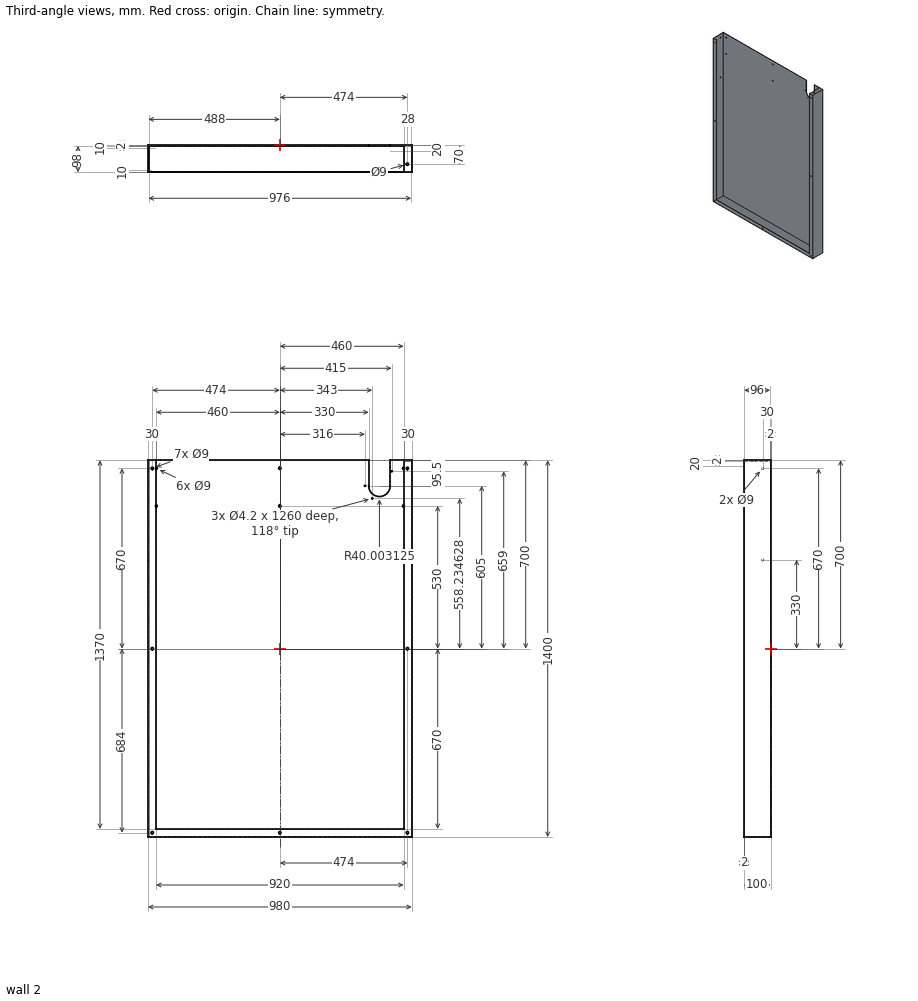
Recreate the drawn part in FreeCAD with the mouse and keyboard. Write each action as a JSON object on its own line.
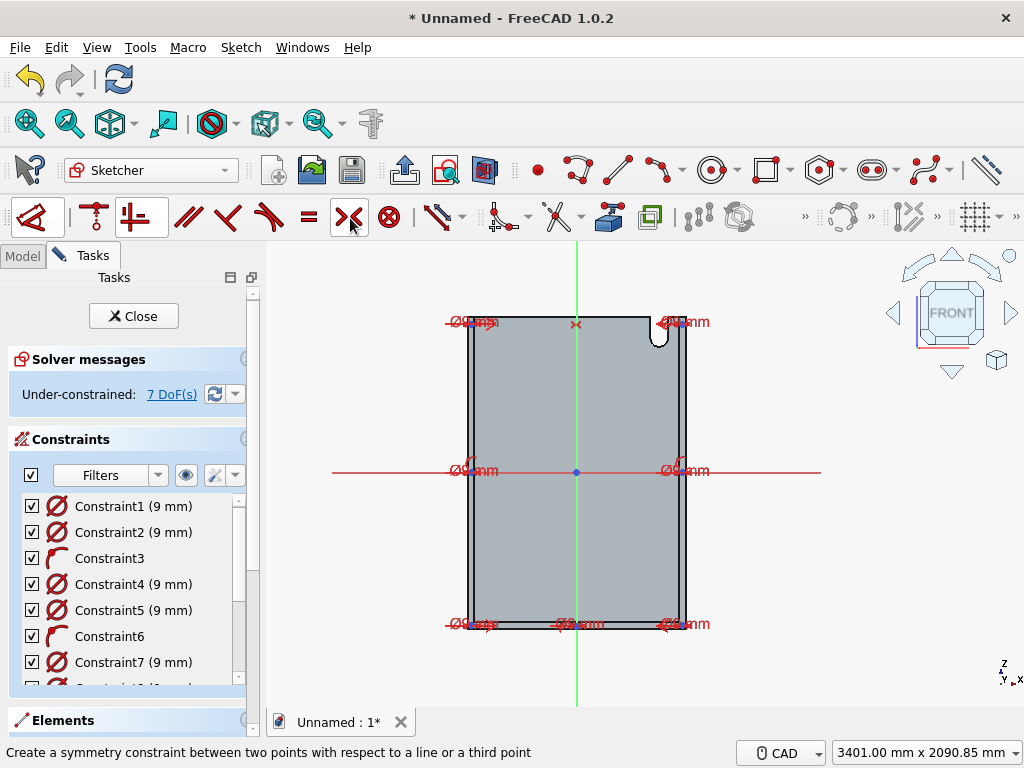
{"action": "left_click", "coordinate": [471, 324]}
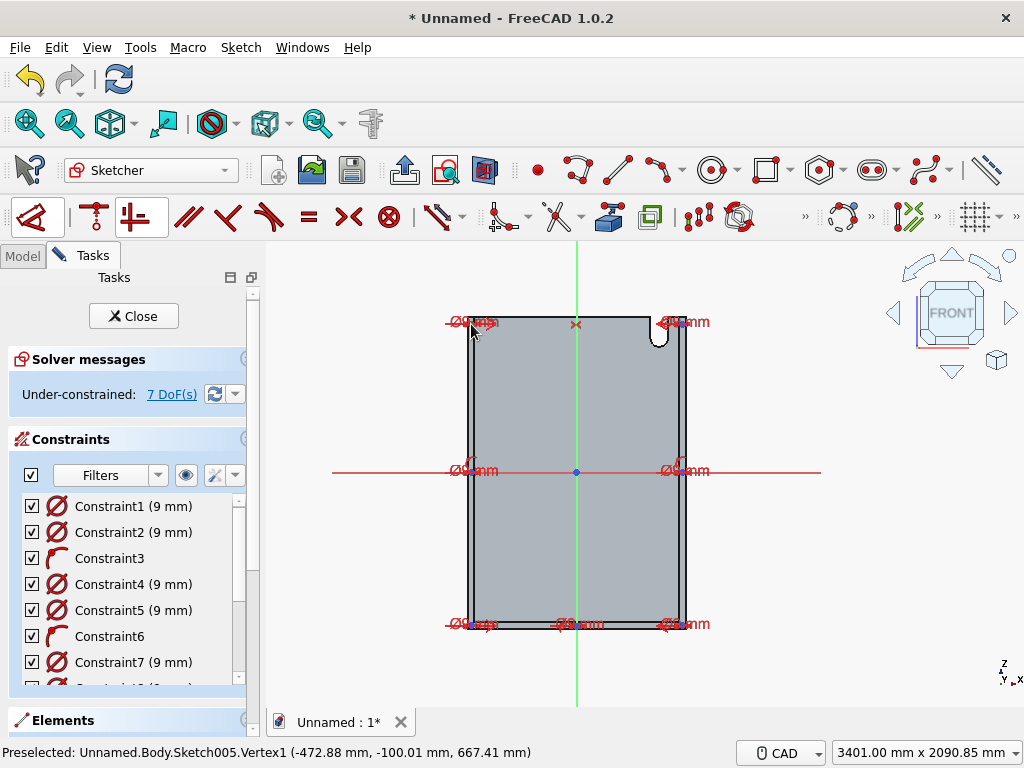
{"action": "key", "text": "l"}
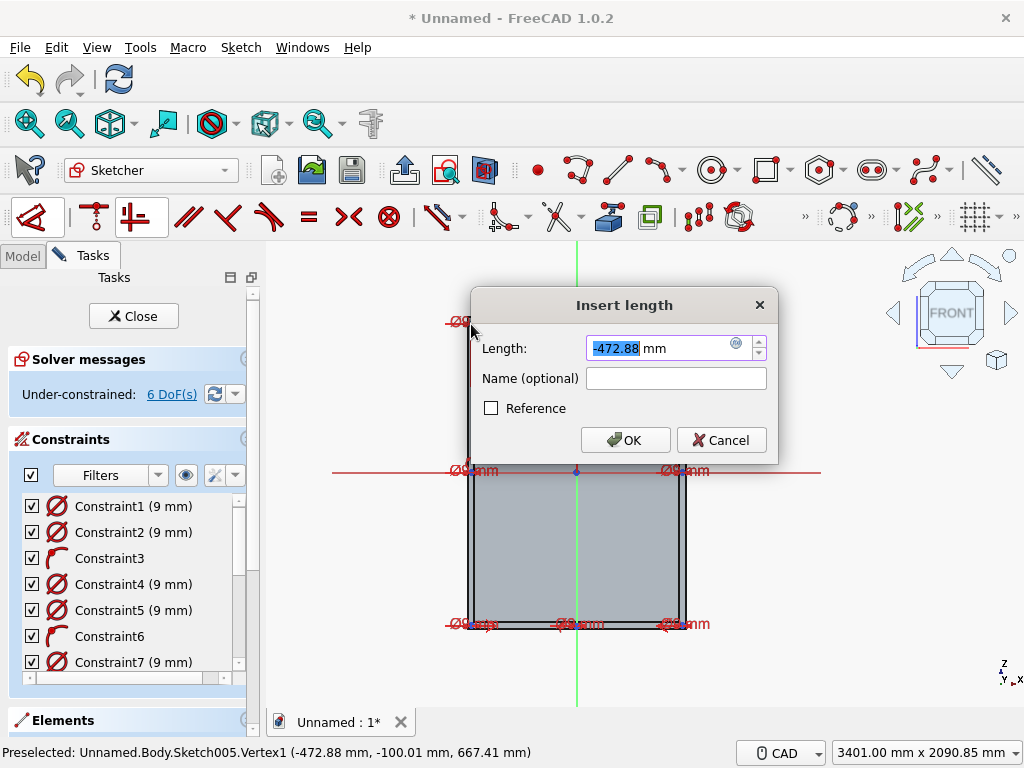
{"action": "type", "text": "-474"}
{"action": "key", "text": "Return"}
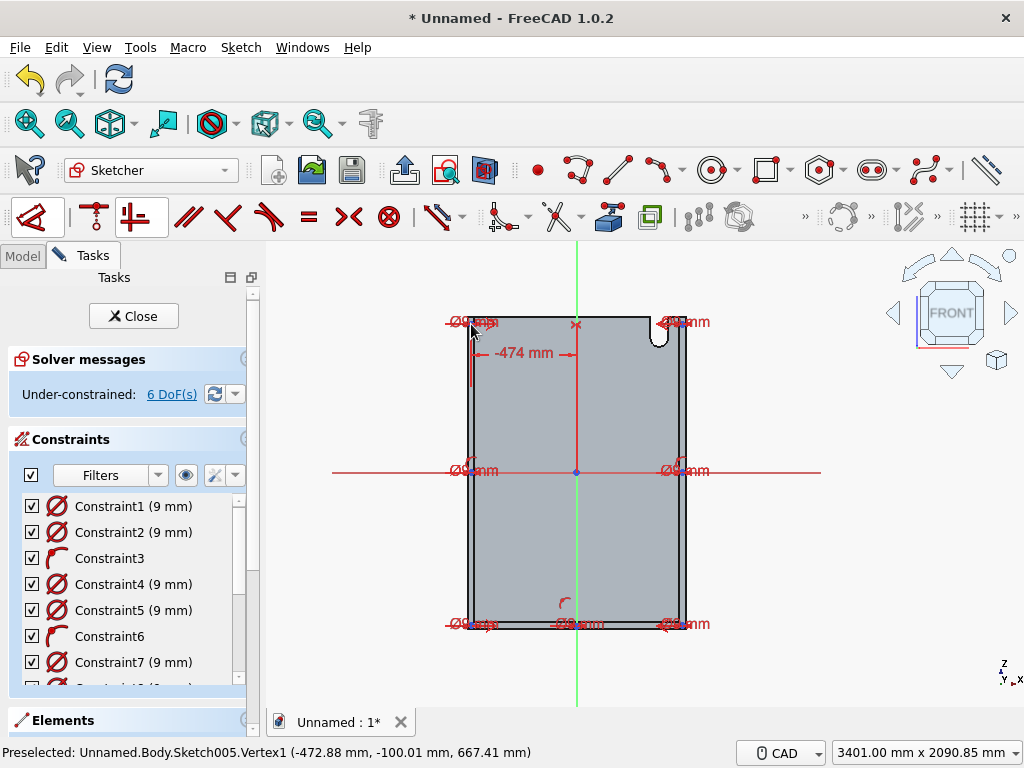
{"action": "left_click", "coordinate": [471, 324]}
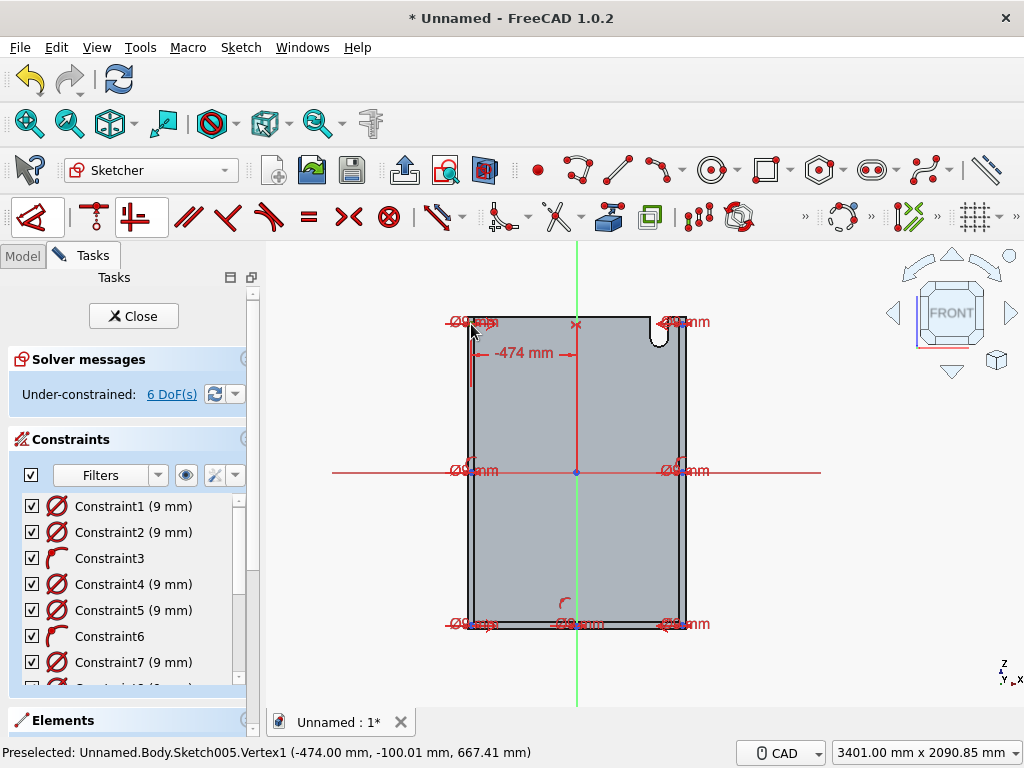
{"action": "key", "text": "i"}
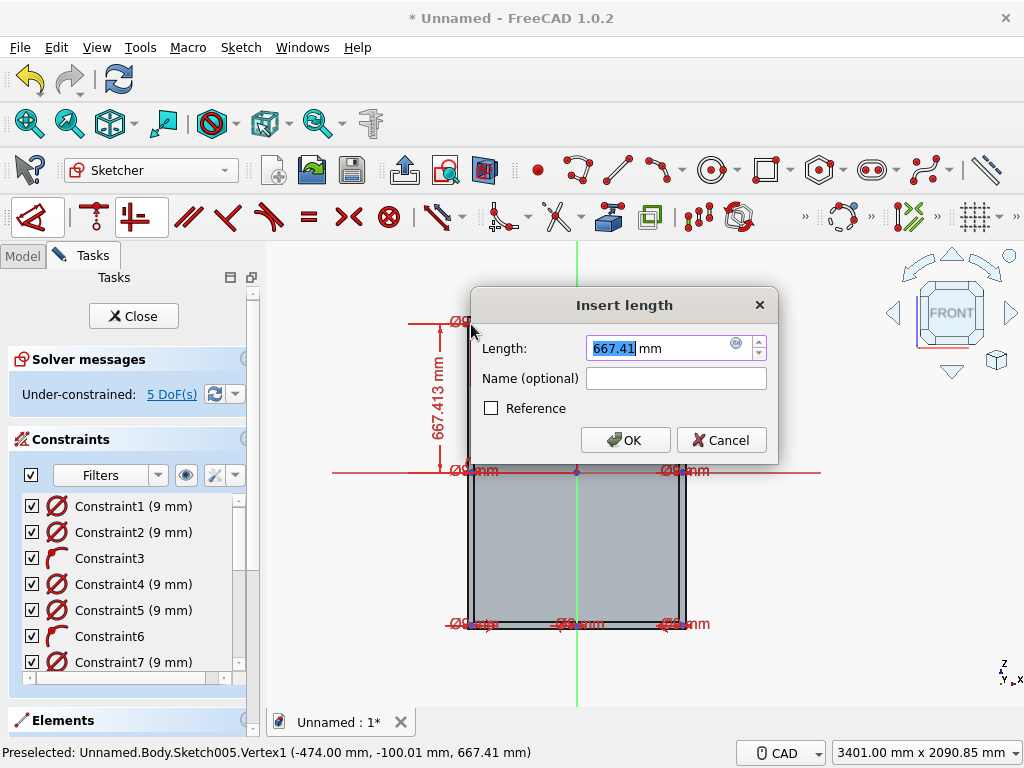
{"action": "type", "text": "670"}
{"action": "key", "text": "Return"}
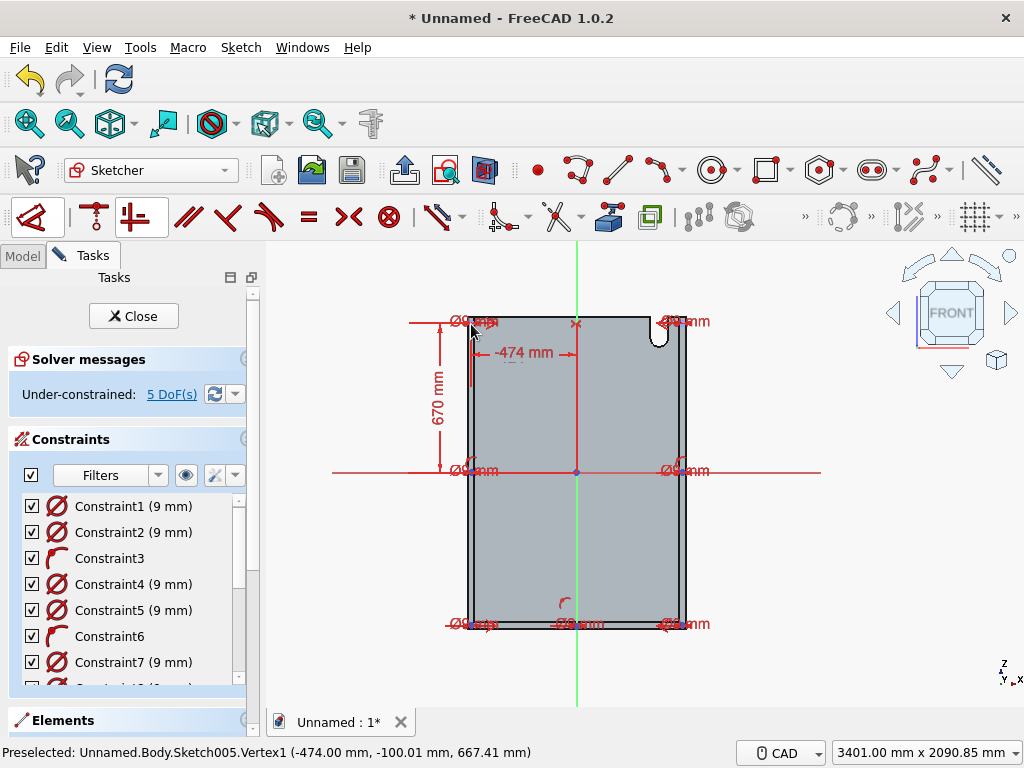
{"action": "left_click", "coordinate": [471, 473]}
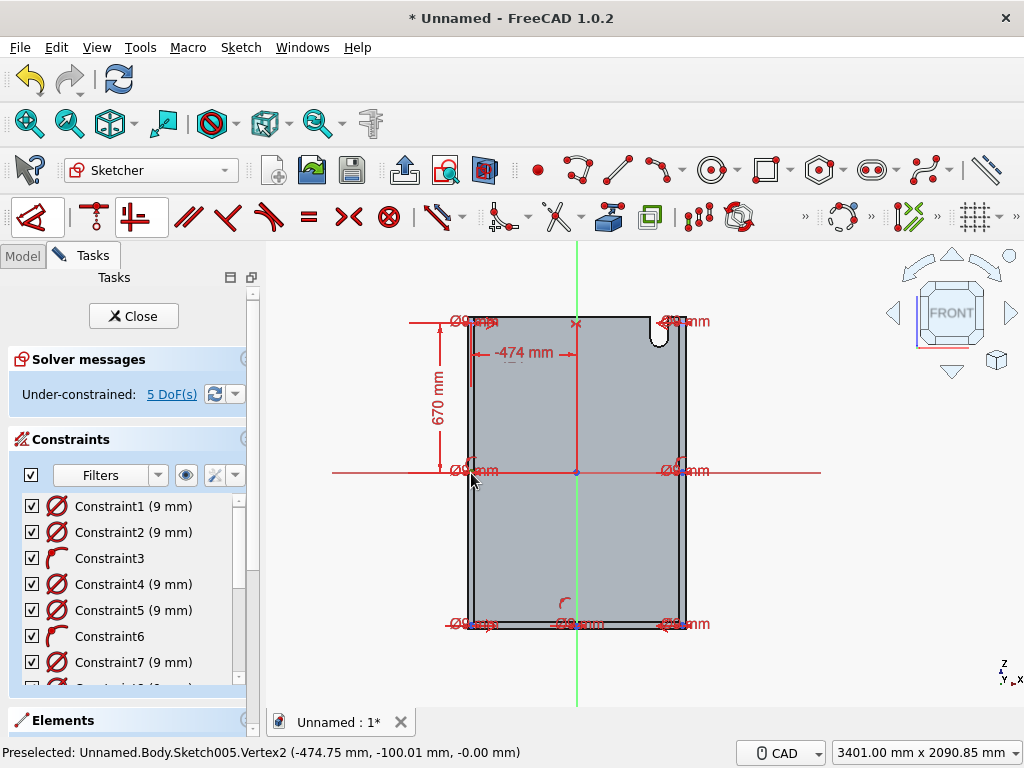
{"action": "key", "text": "l"}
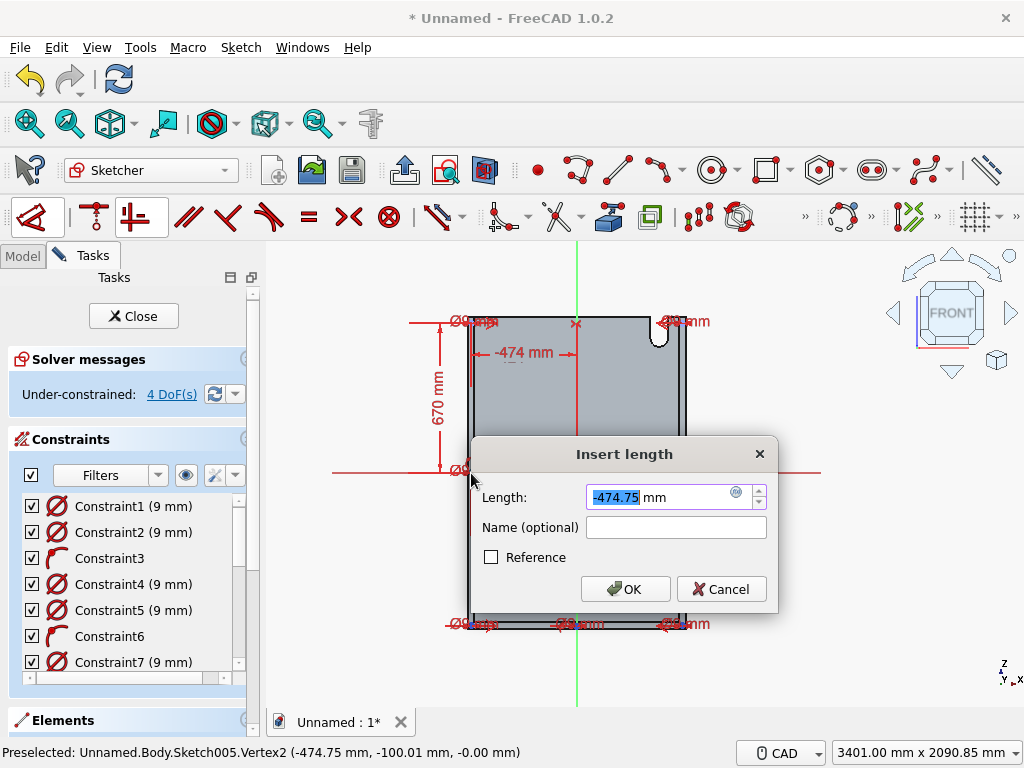
{"action": "type", "text": "-474"}
{"action": "key", "text": "Return"}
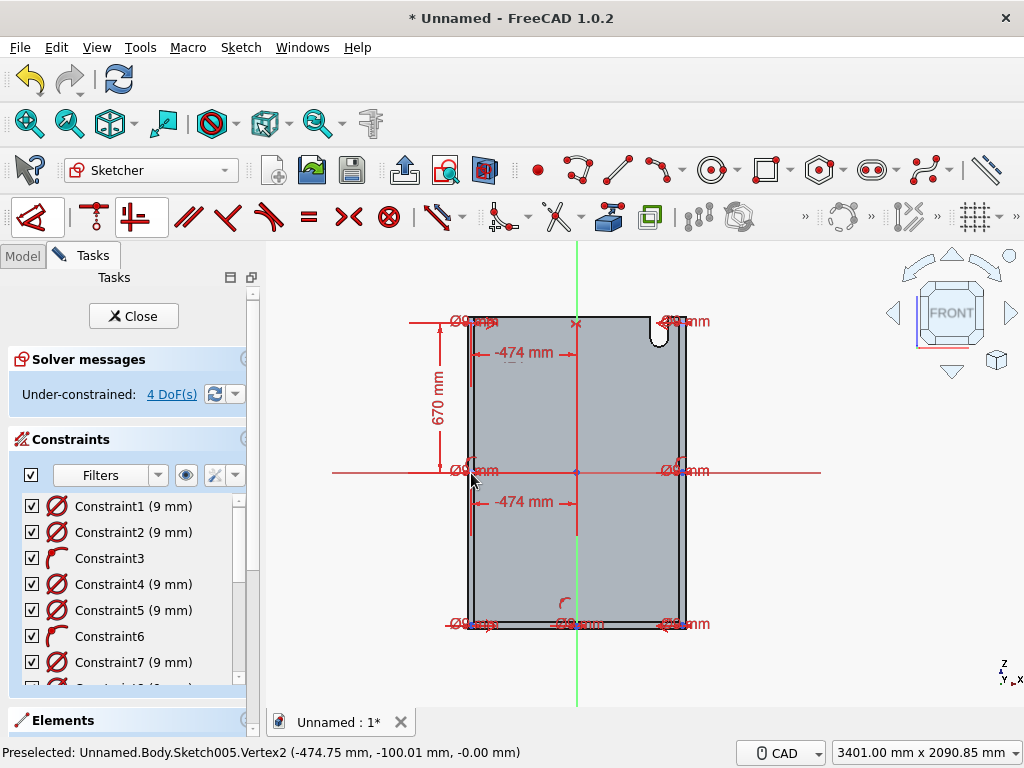
{"action": "left_click", "coordinate": [471, 626]}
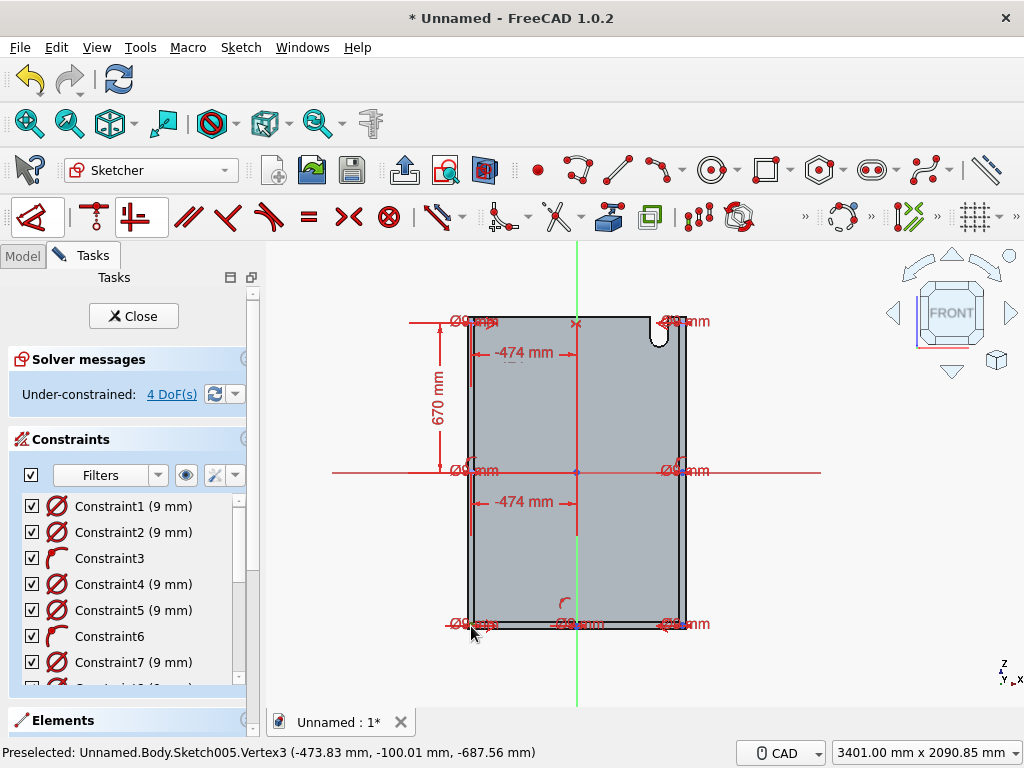
{"action": "key", "text": "l"}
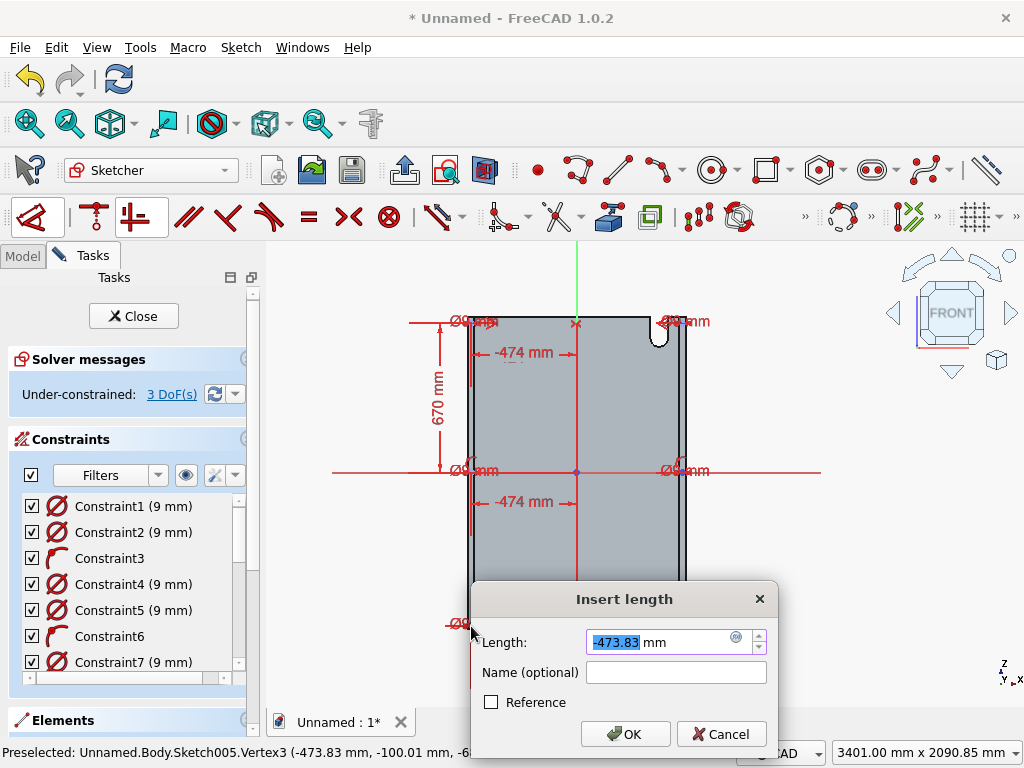
{"action": "type", "text": "-474"}
{"action": "key", "text": "Return"}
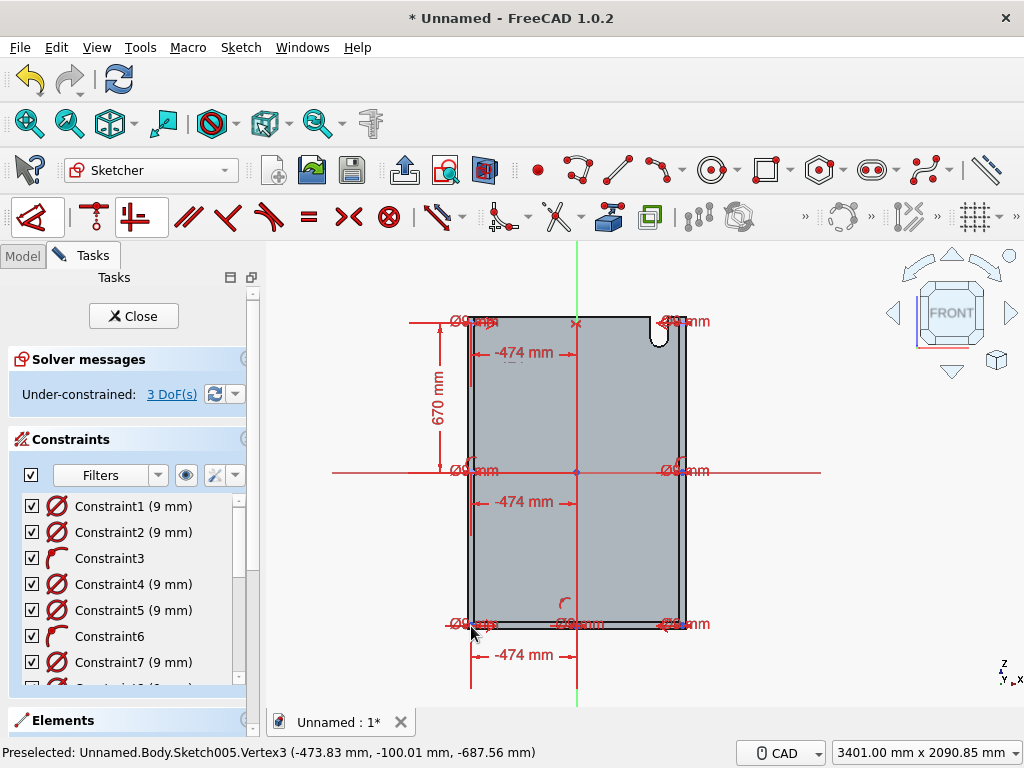
{"action": "left_click", "coordinate": [471, 626]}